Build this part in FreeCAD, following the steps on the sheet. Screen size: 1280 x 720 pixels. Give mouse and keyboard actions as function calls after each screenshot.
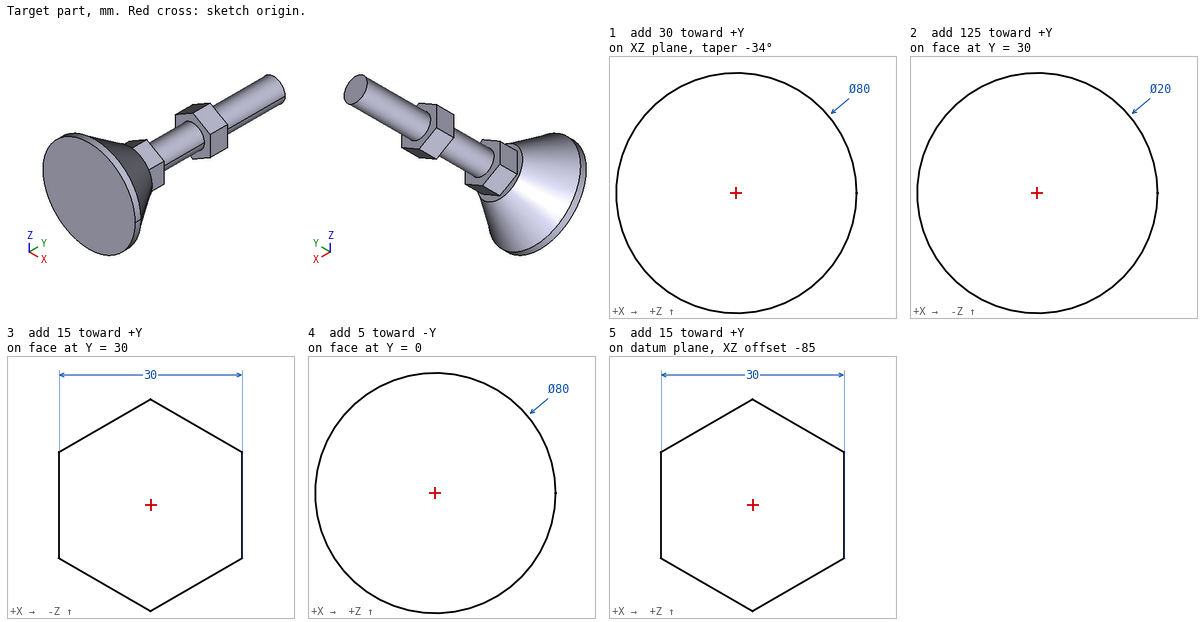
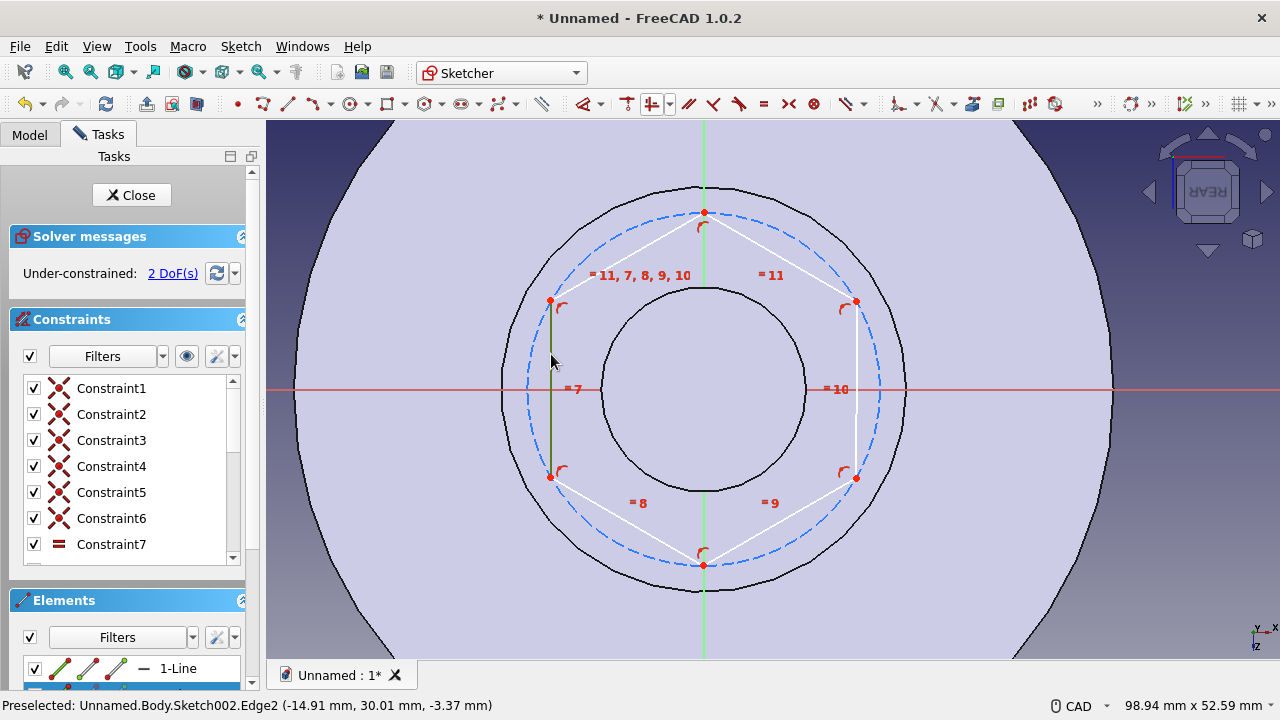
key(v)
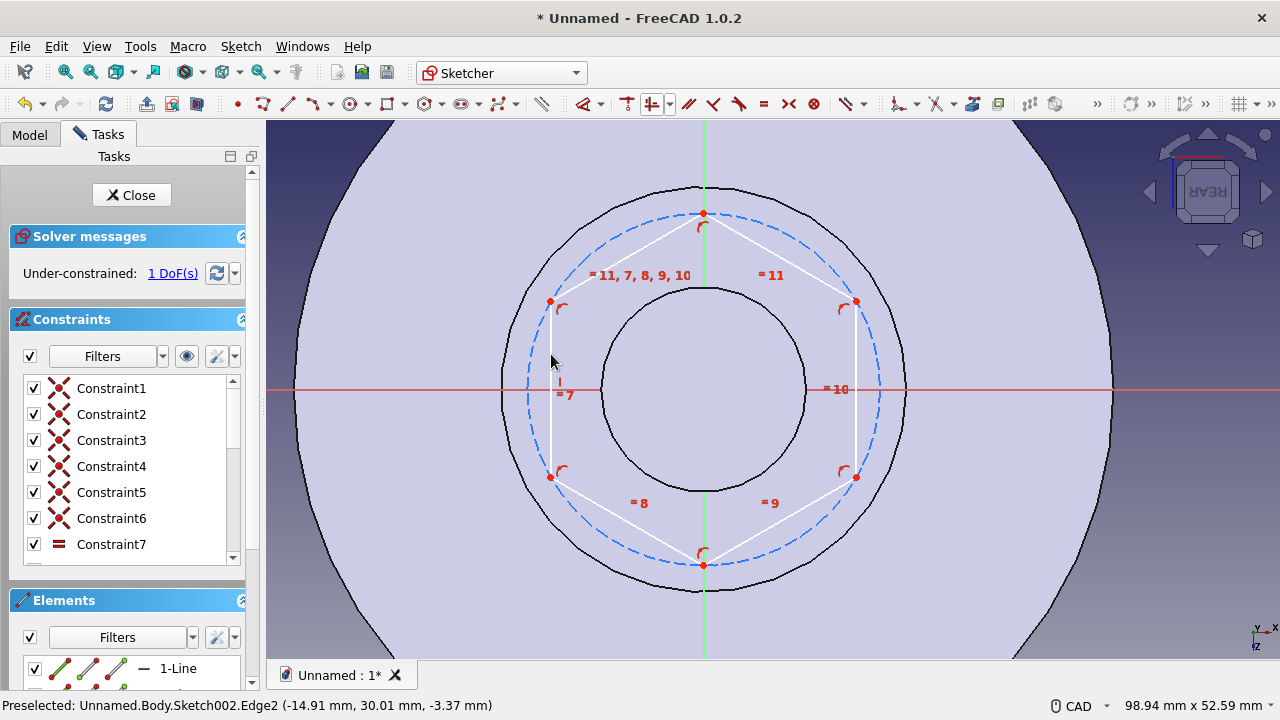
click(582, 104)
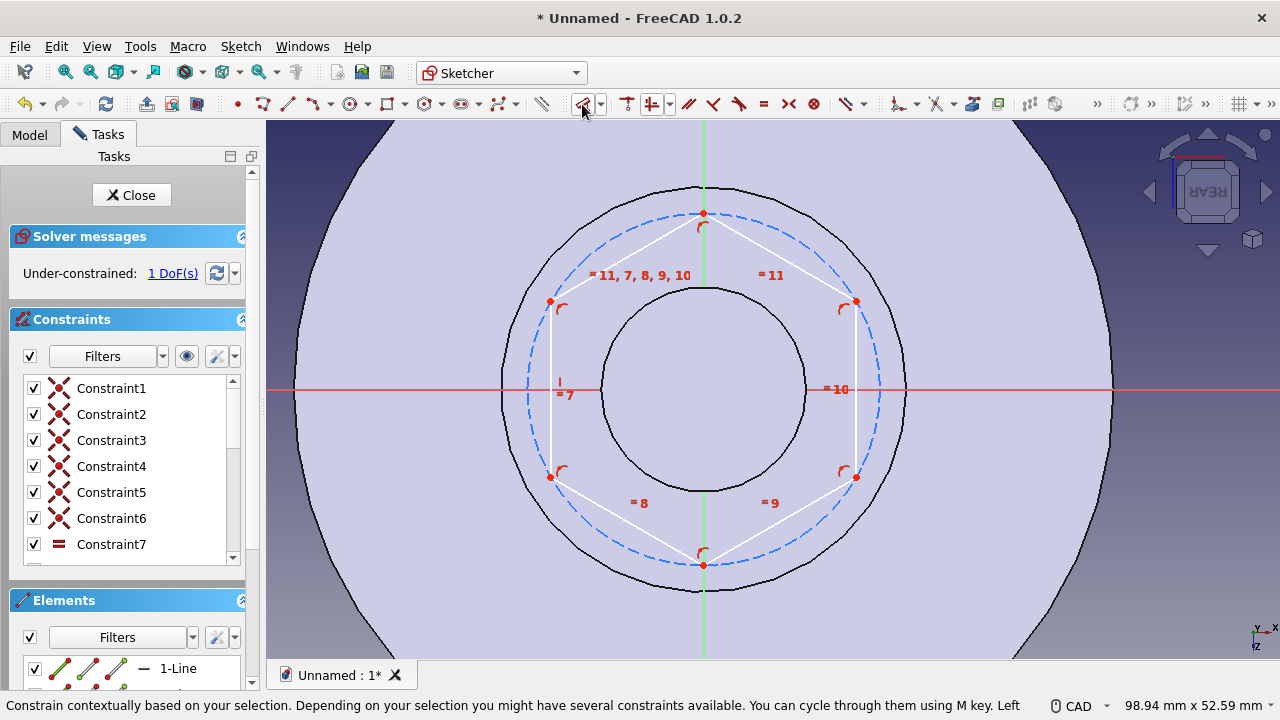
click(551, 301)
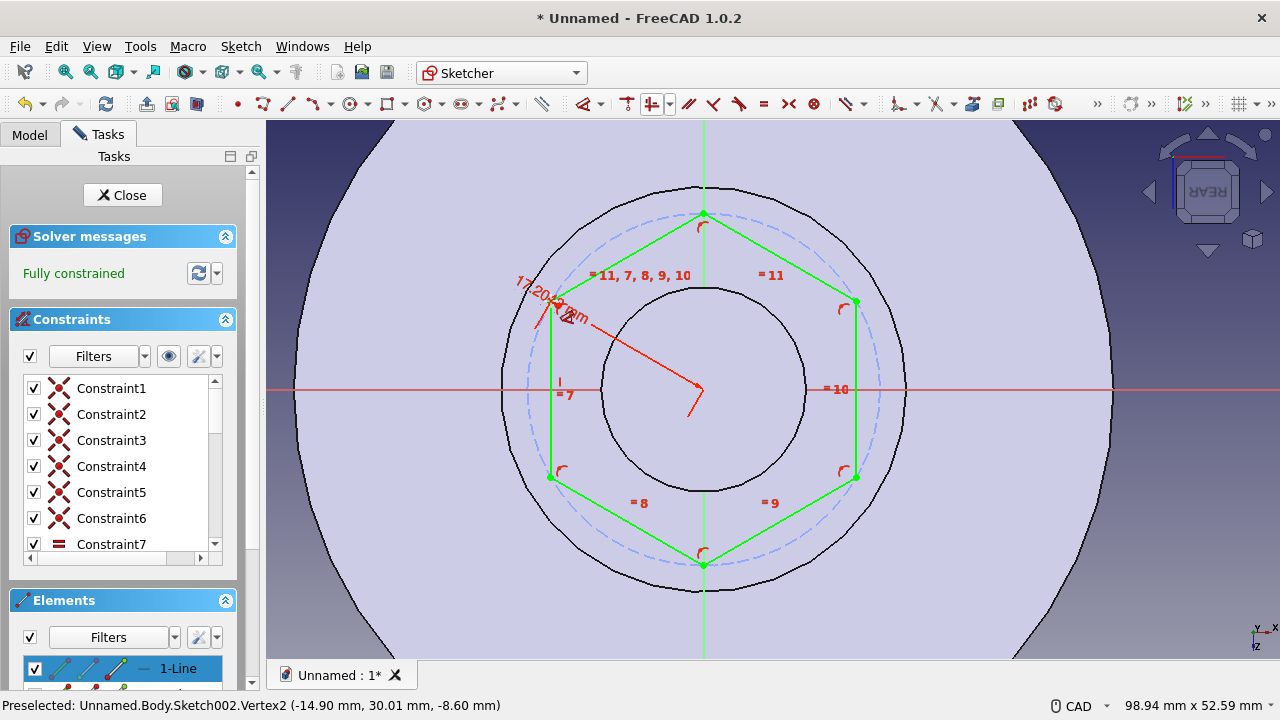
click(856, 478)
click(597, 560)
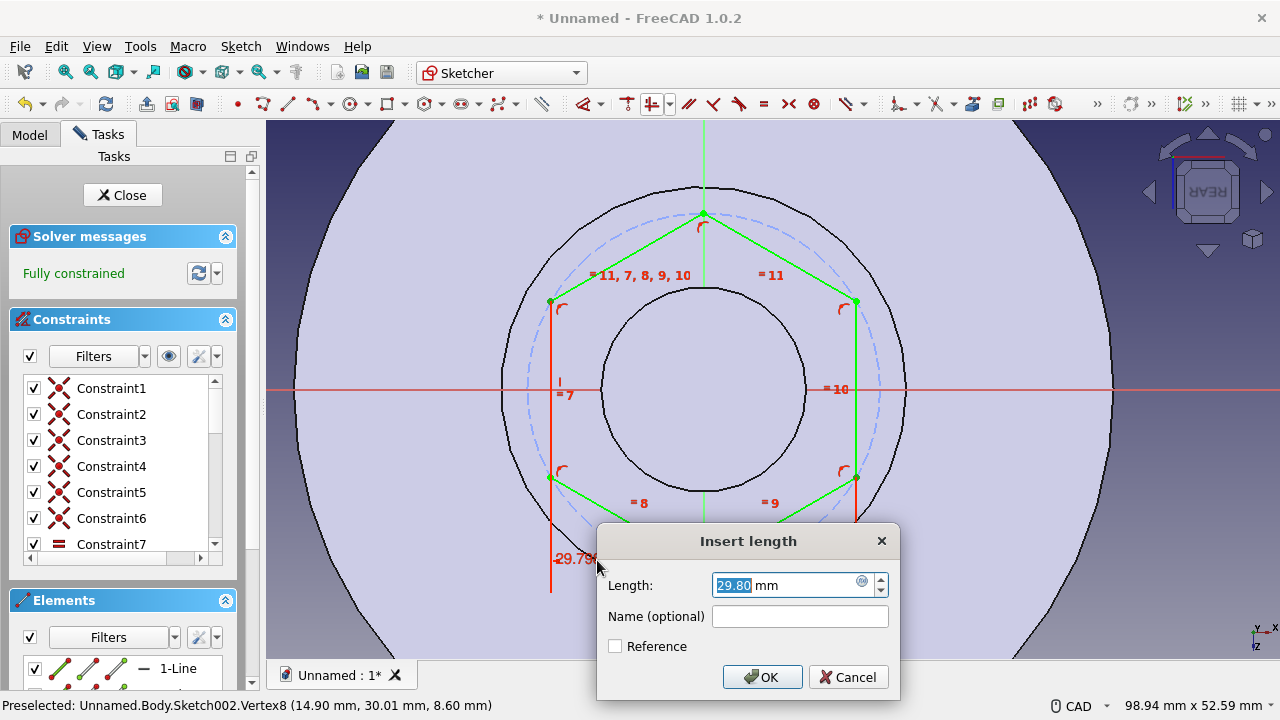
text(30)
key(Return)
key(Escape)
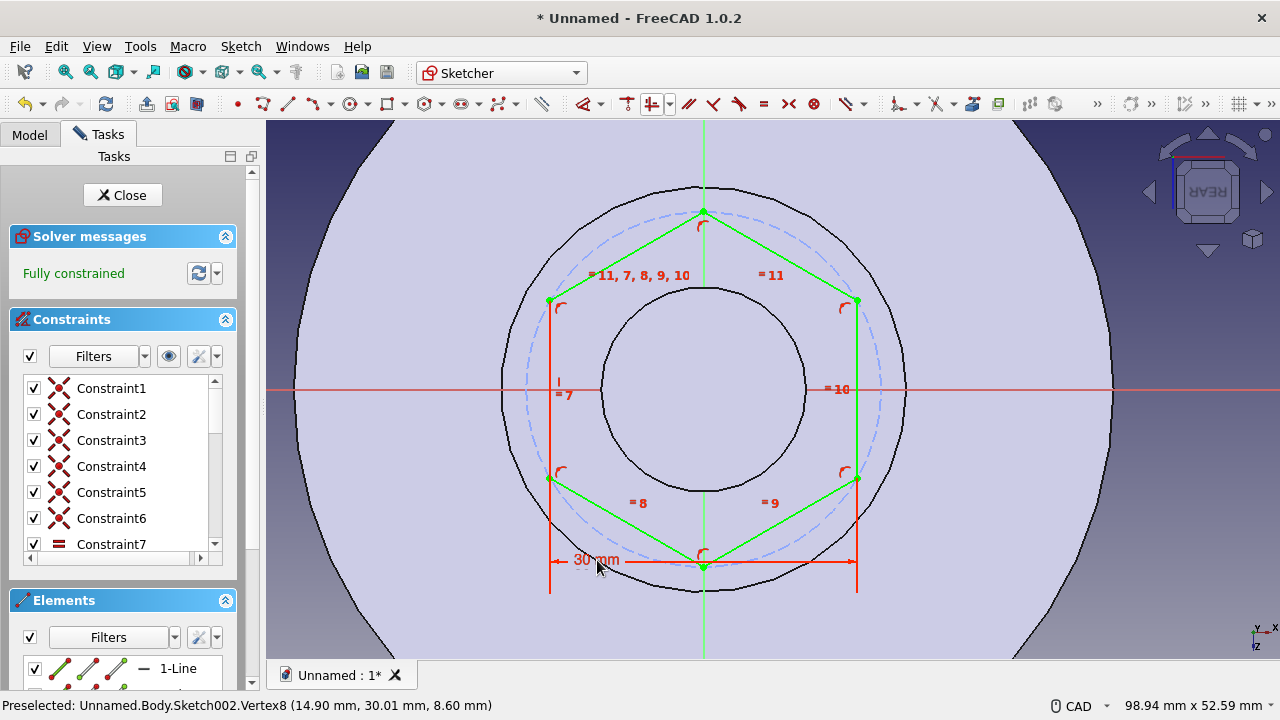
click(123, 195)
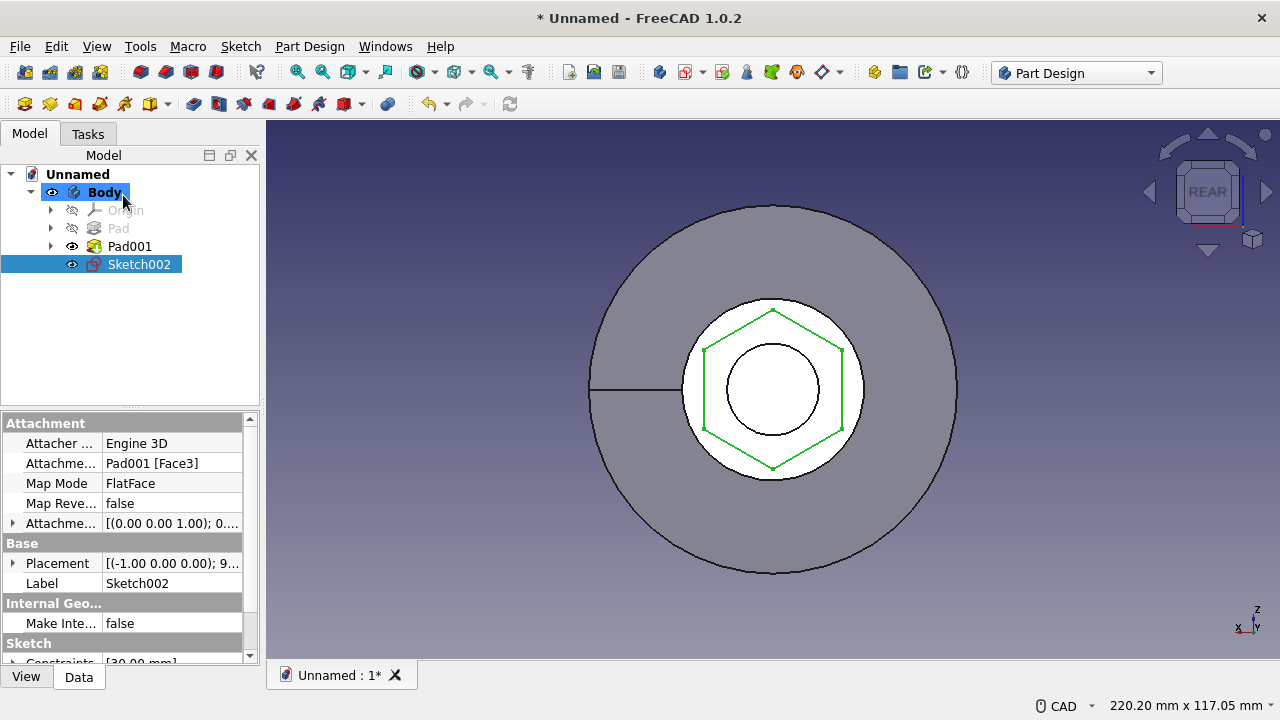
click(25, 104)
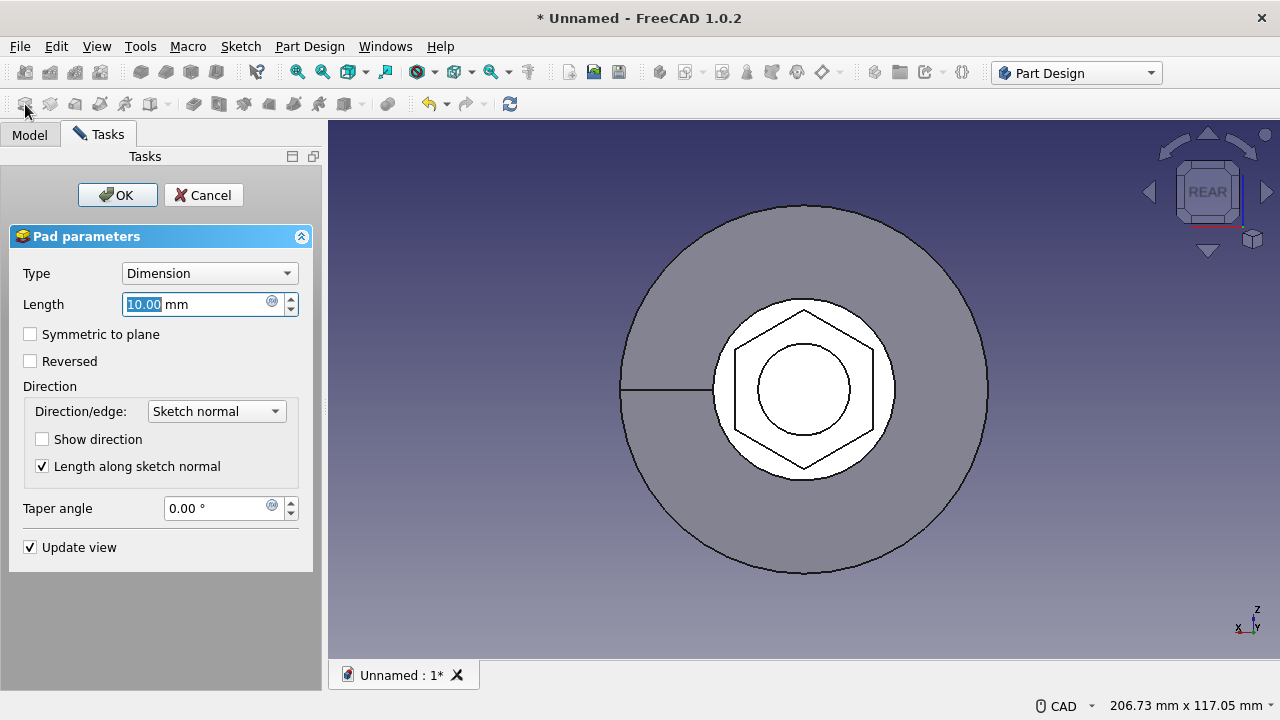
text(15)
key(Tab)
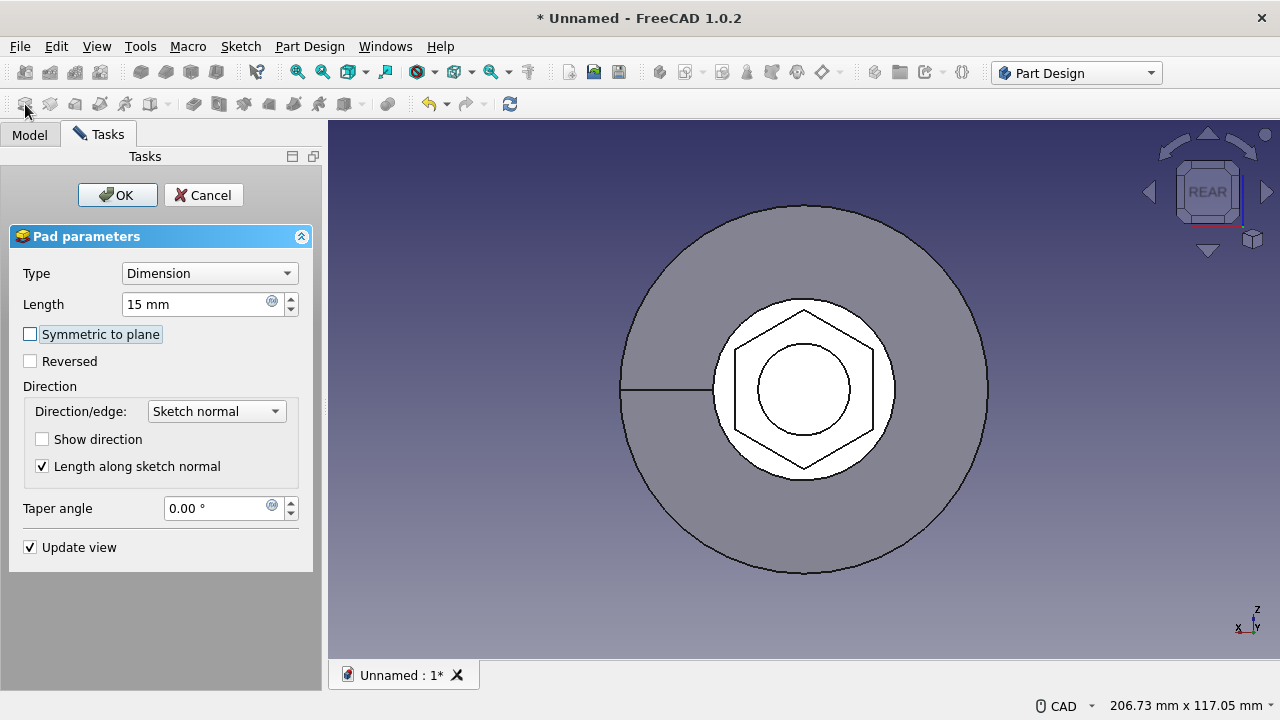
click(118, 195)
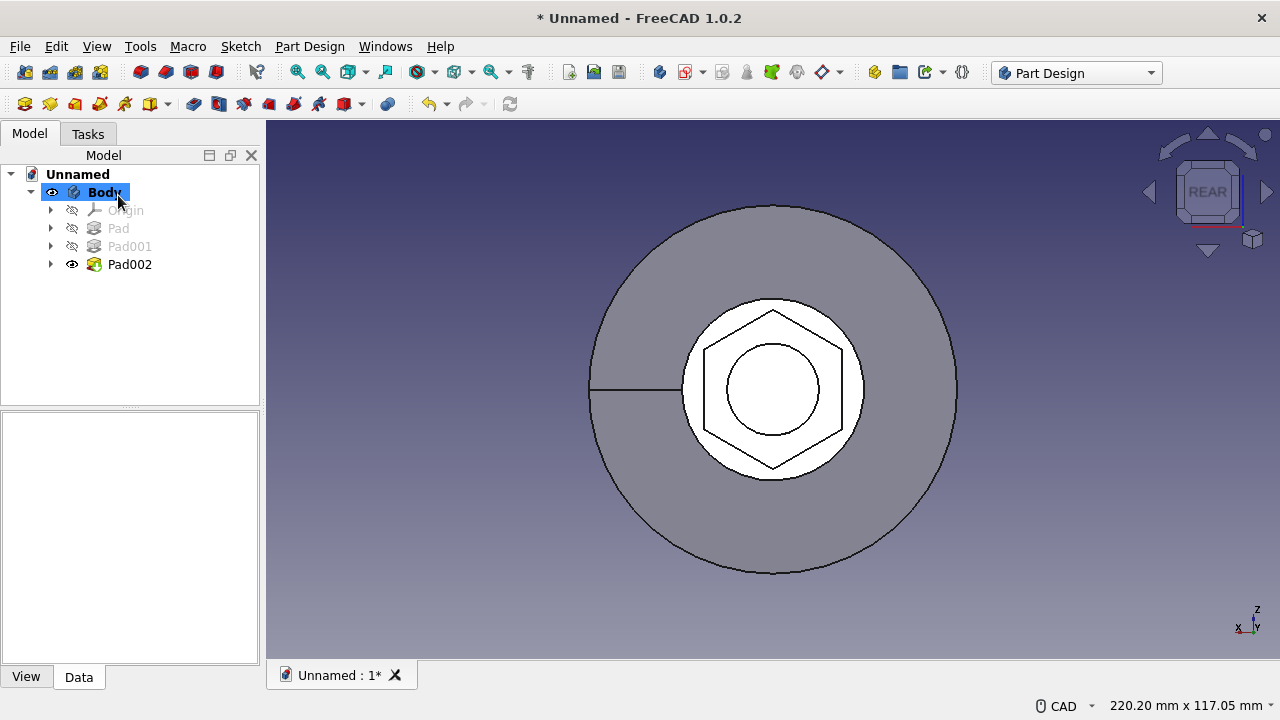
key(0)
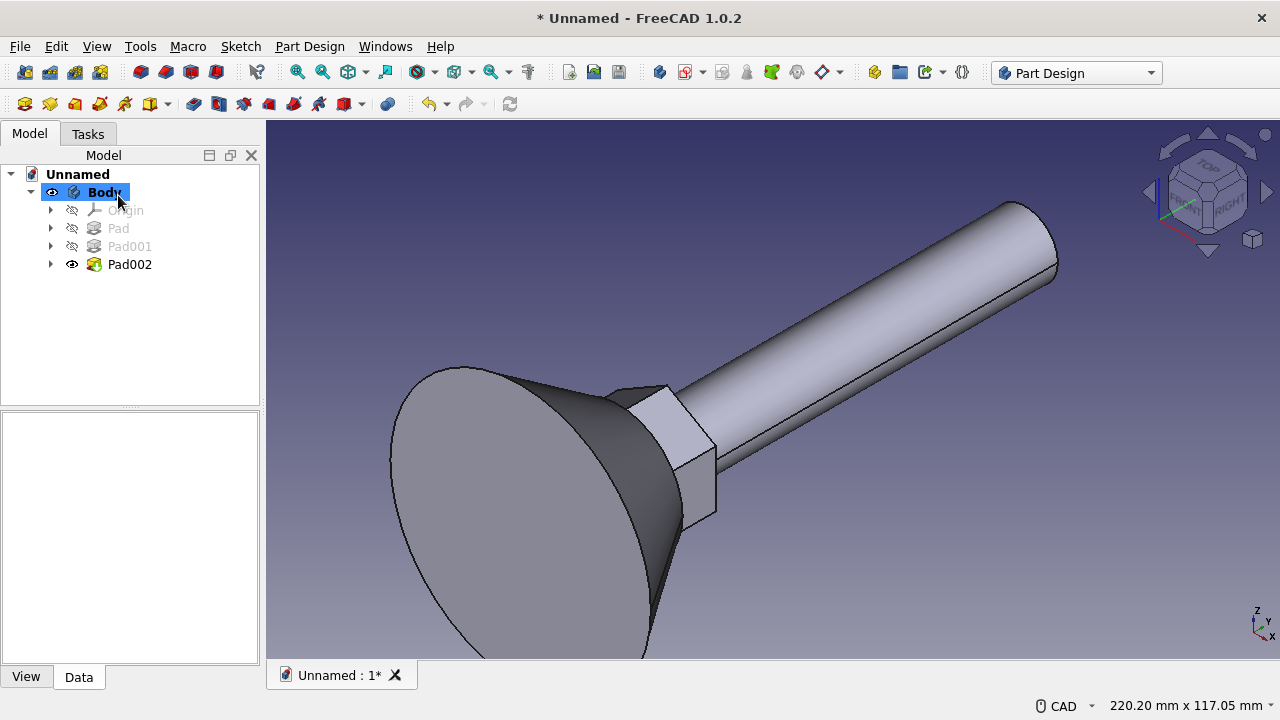
click(298, 72)